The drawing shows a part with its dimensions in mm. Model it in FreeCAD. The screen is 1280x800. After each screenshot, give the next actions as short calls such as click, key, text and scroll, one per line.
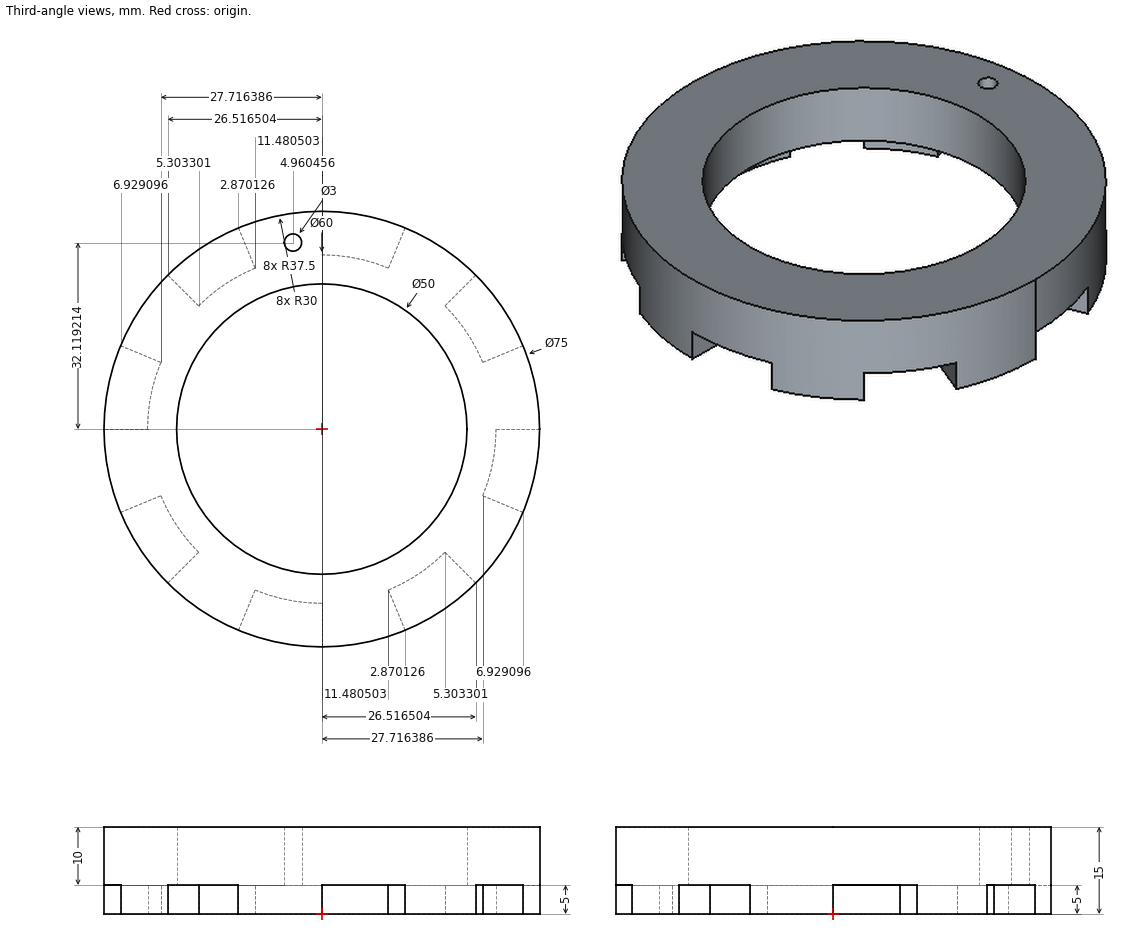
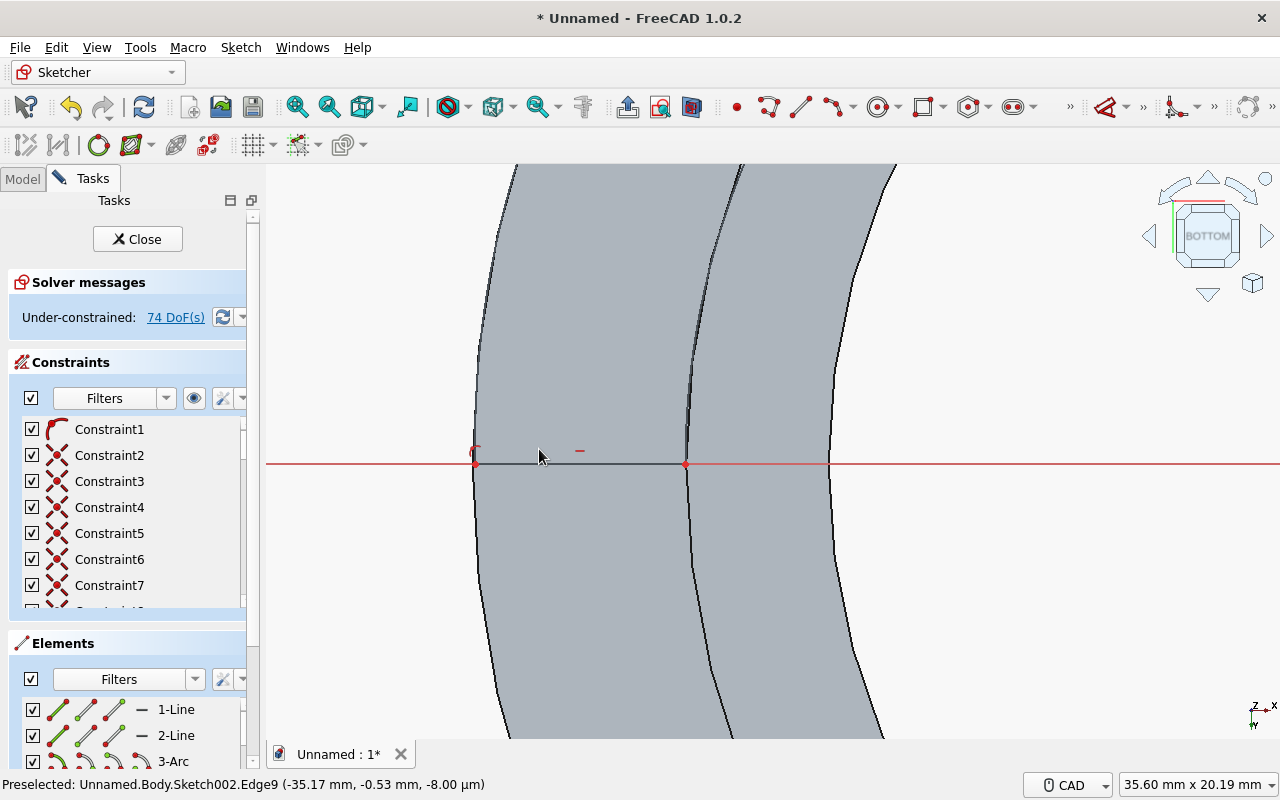
scroll(539, 449, down, 9)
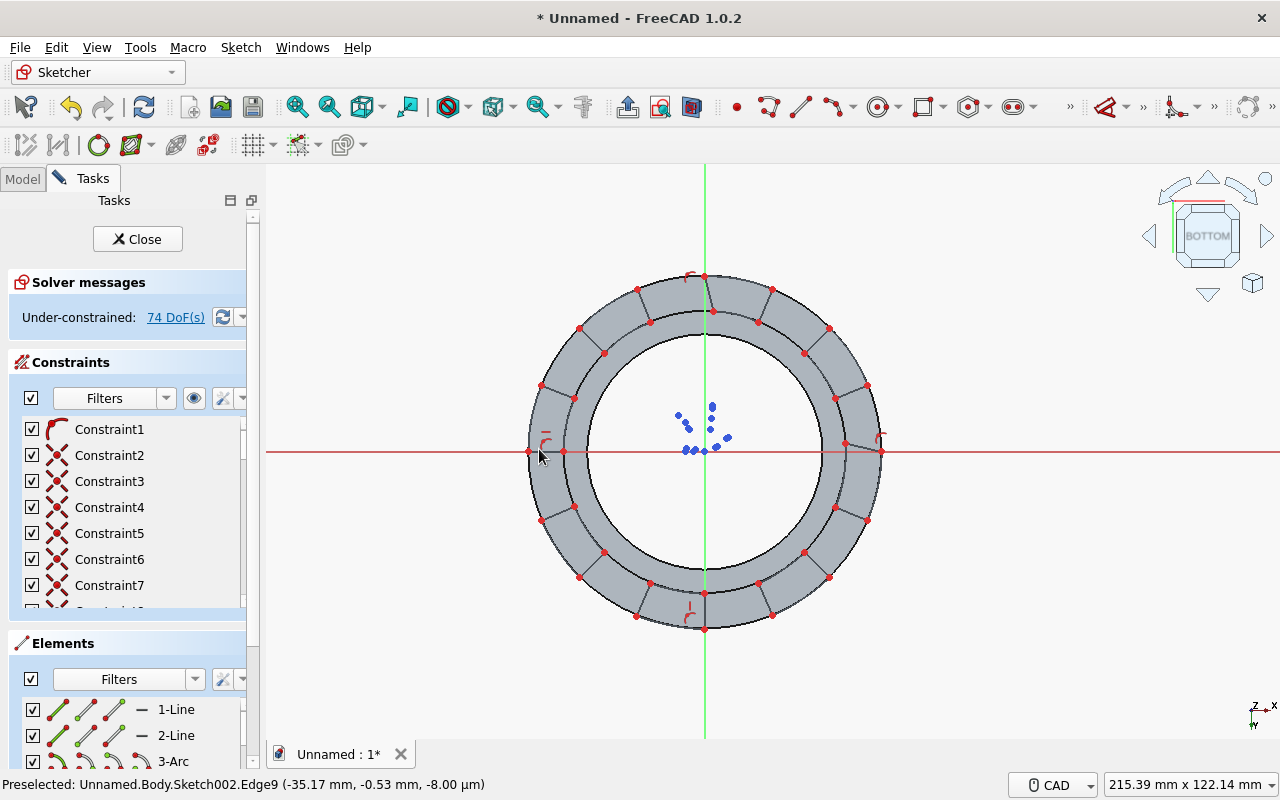
scroll(707, 287, up, 9)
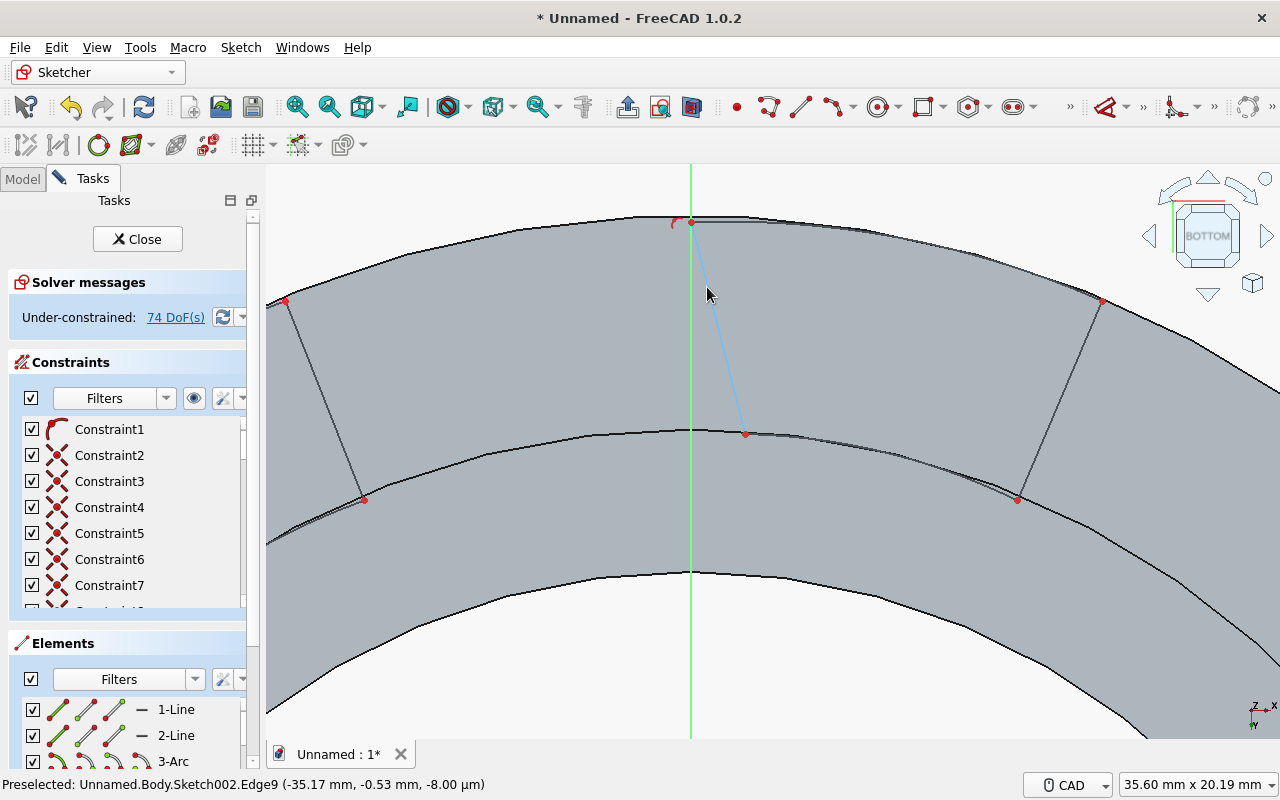
click(708, 286)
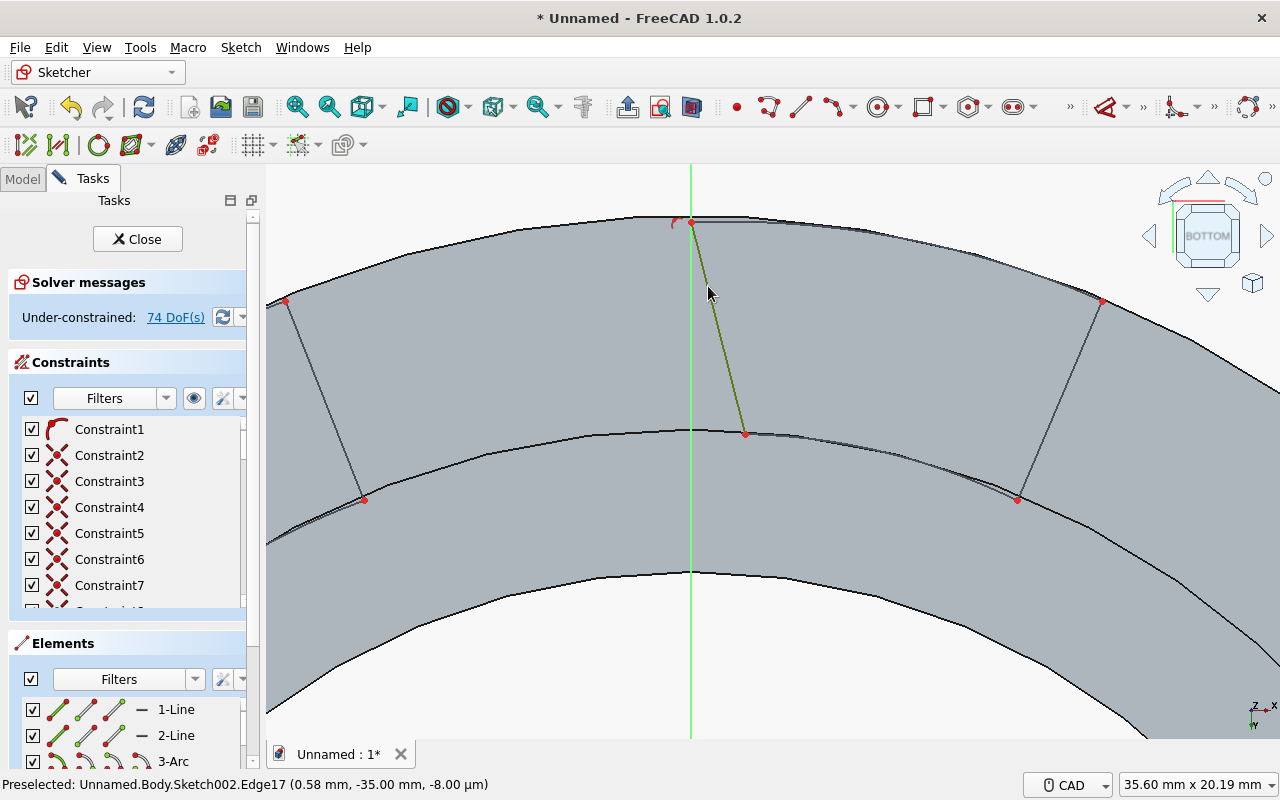
key(v)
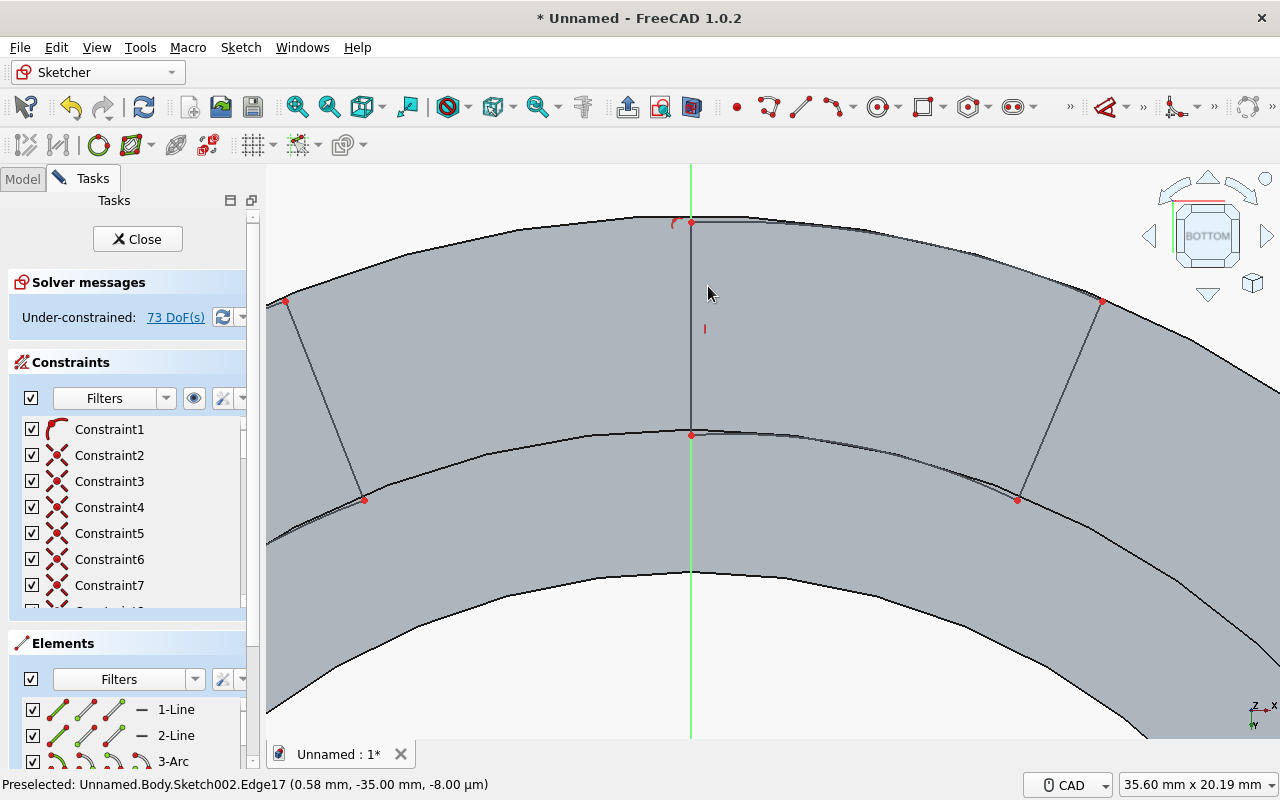
scroll(707, 287, down, 9)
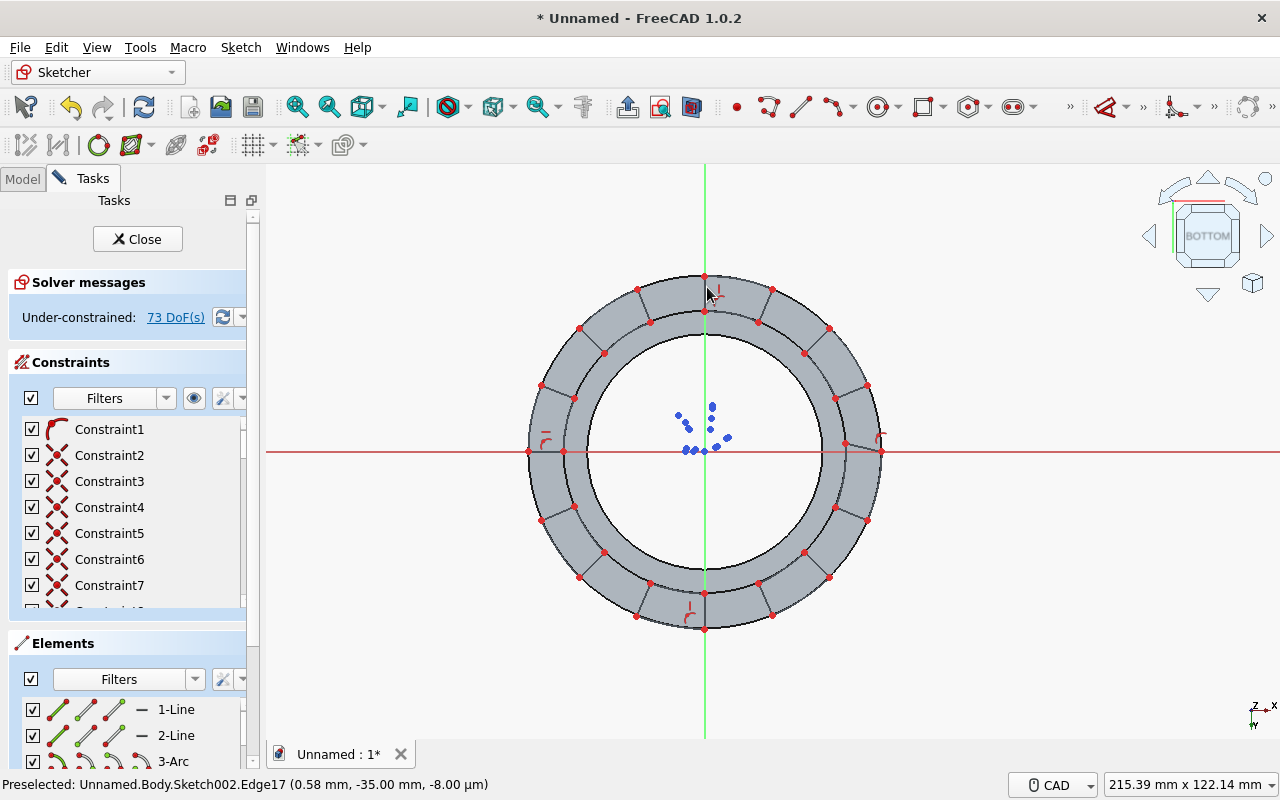
scroll(871, 449, up, 9)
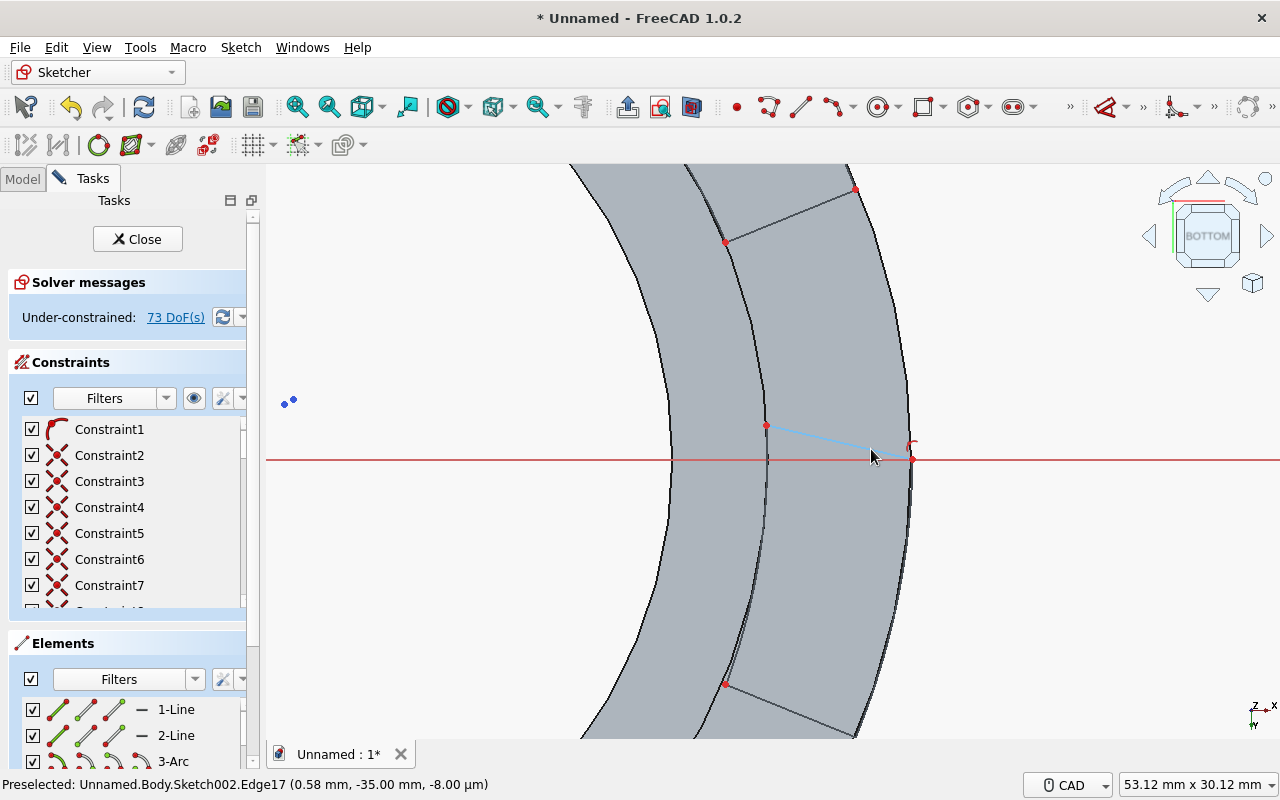
click(867, 449)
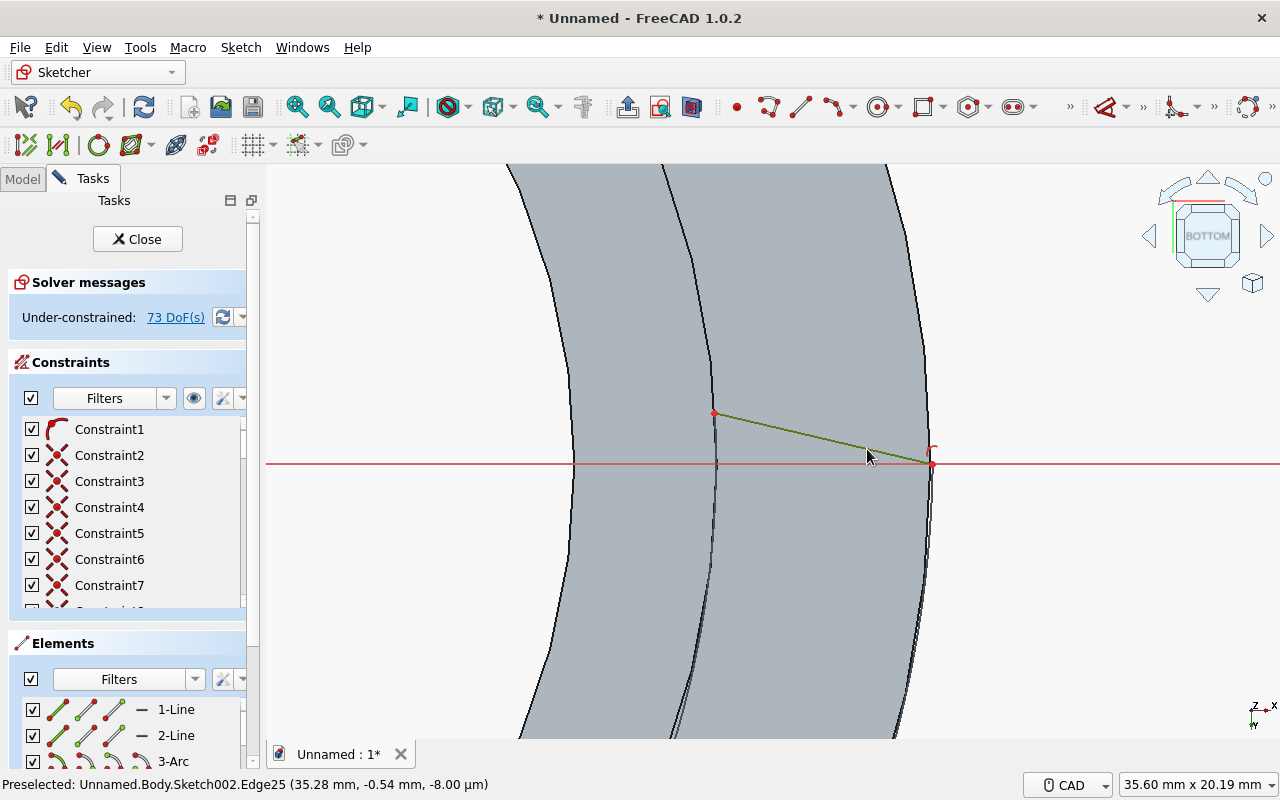
key(h)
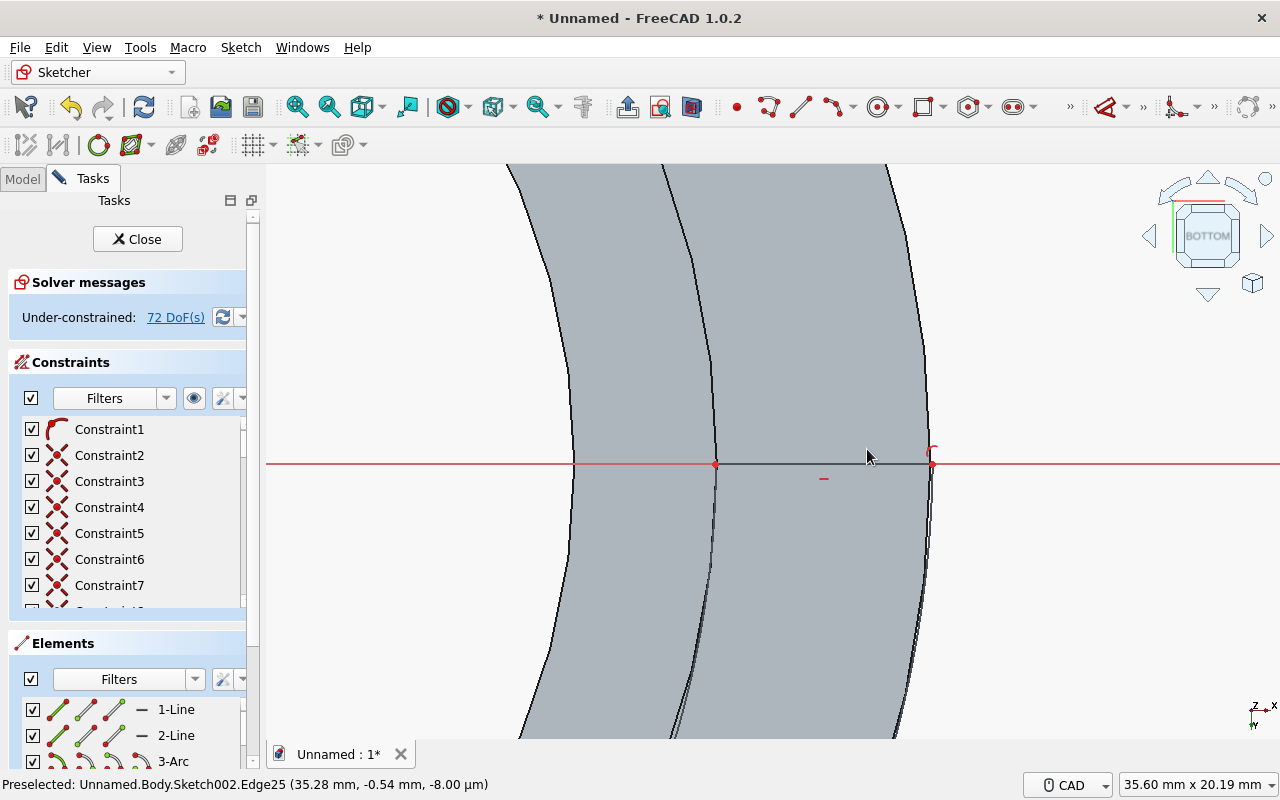
scroll(871, 449, down, 9)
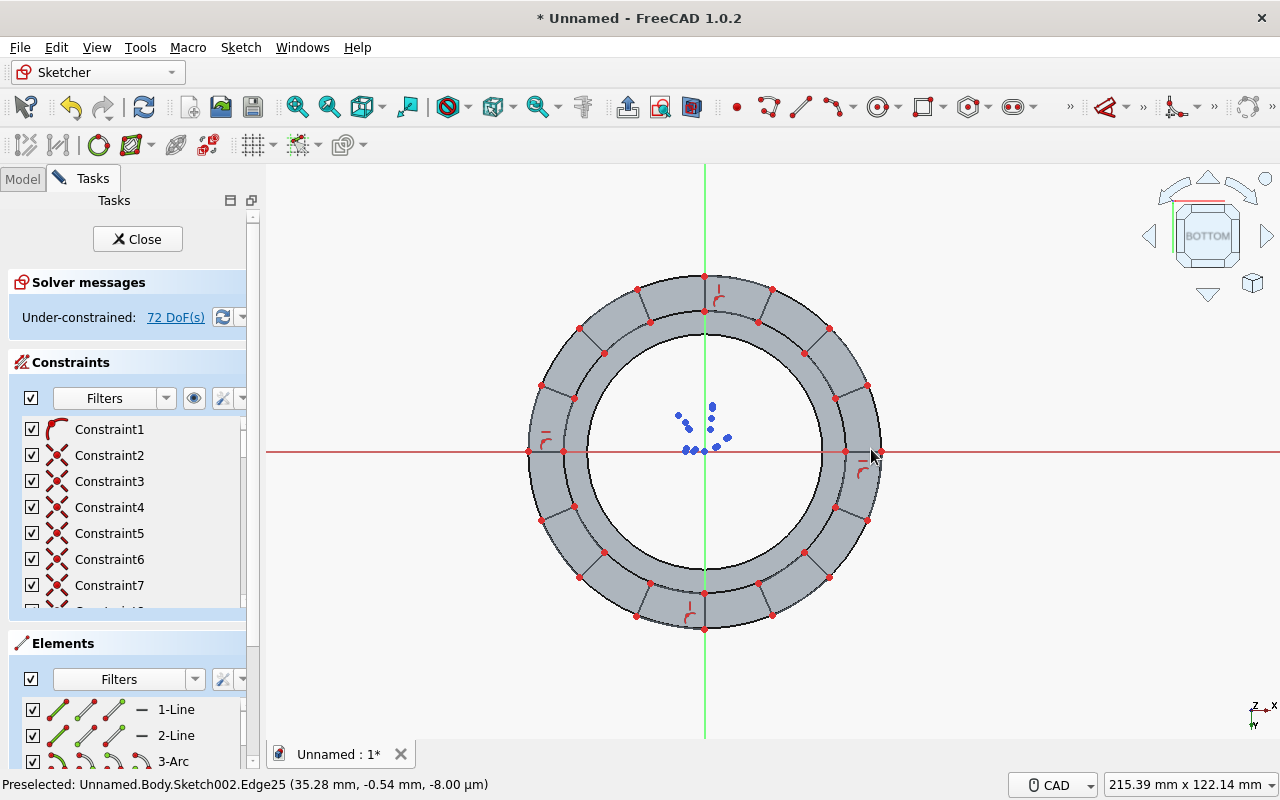
click(667, 588)